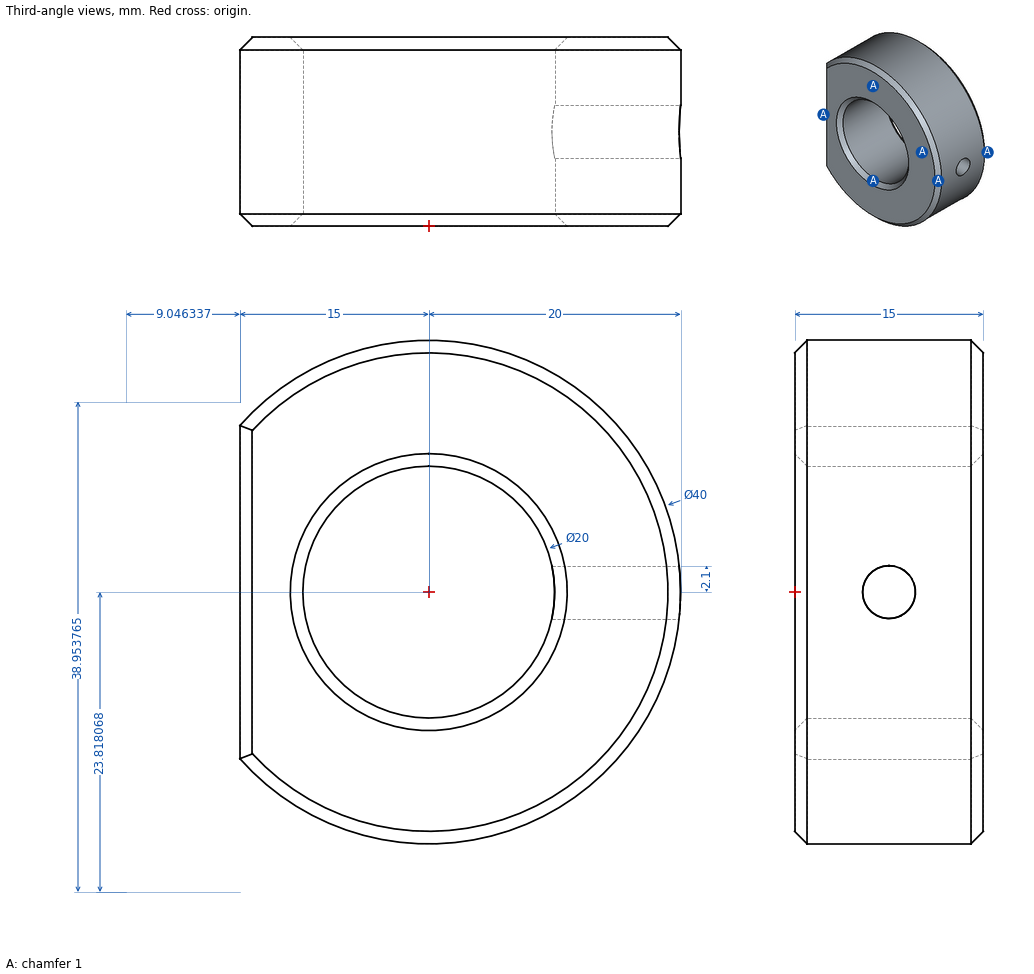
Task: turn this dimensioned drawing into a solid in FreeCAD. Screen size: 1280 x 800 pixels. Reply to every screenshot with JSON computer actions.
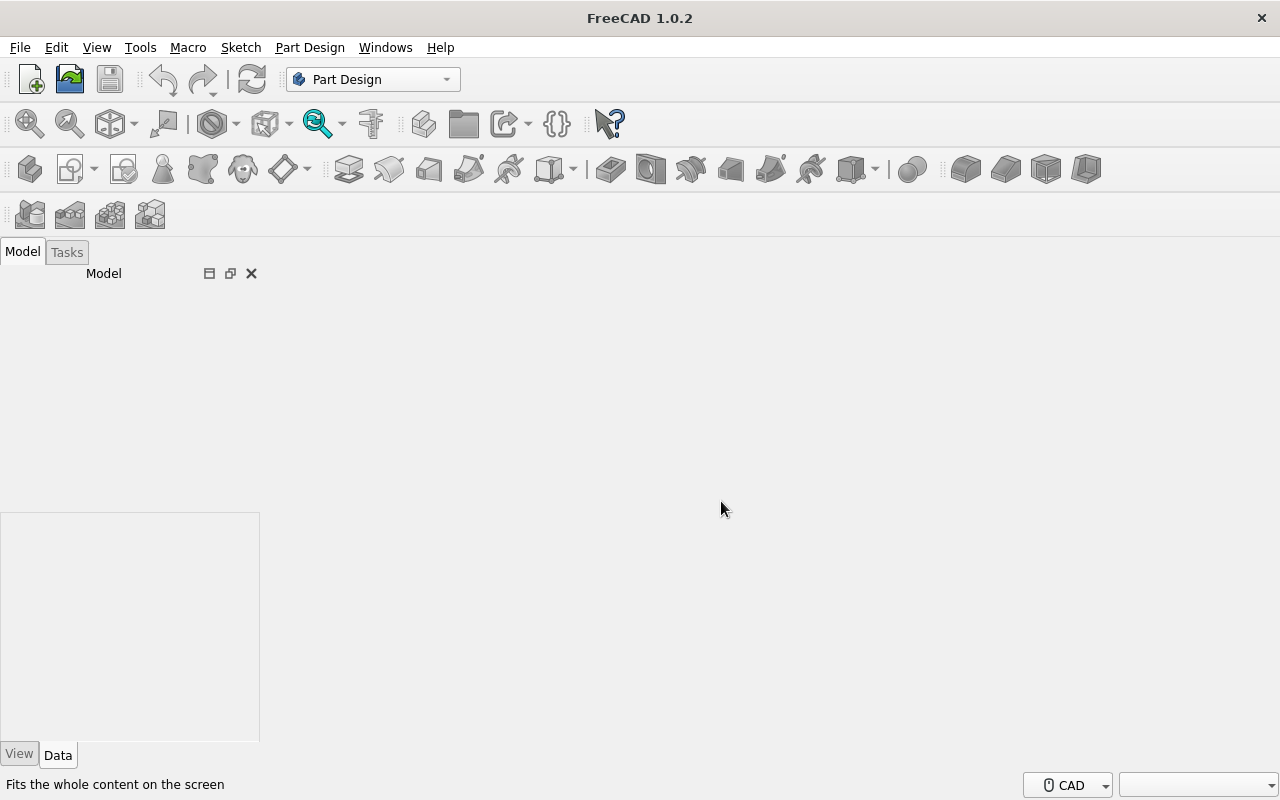
{"action": "key", "text": "ctrl+n"}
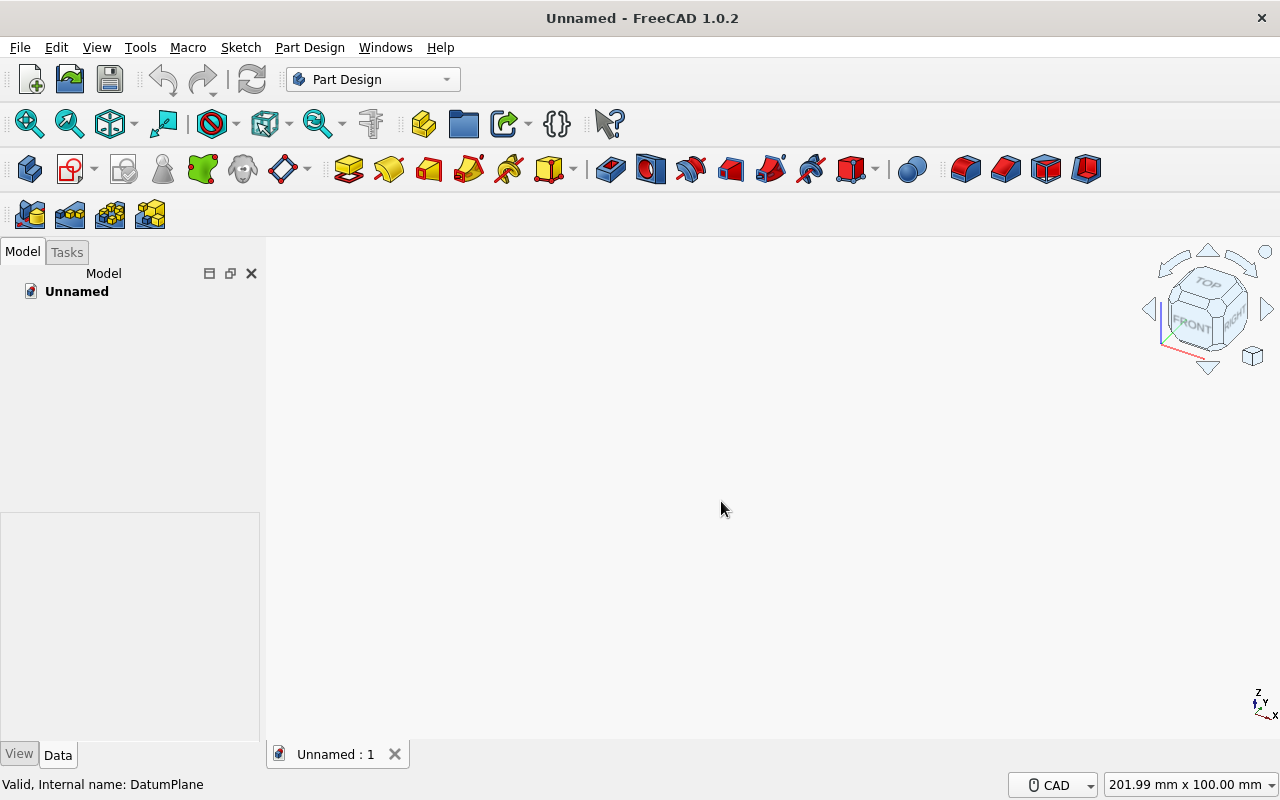
{"action": "left_click", "coordinate": [70, 170]}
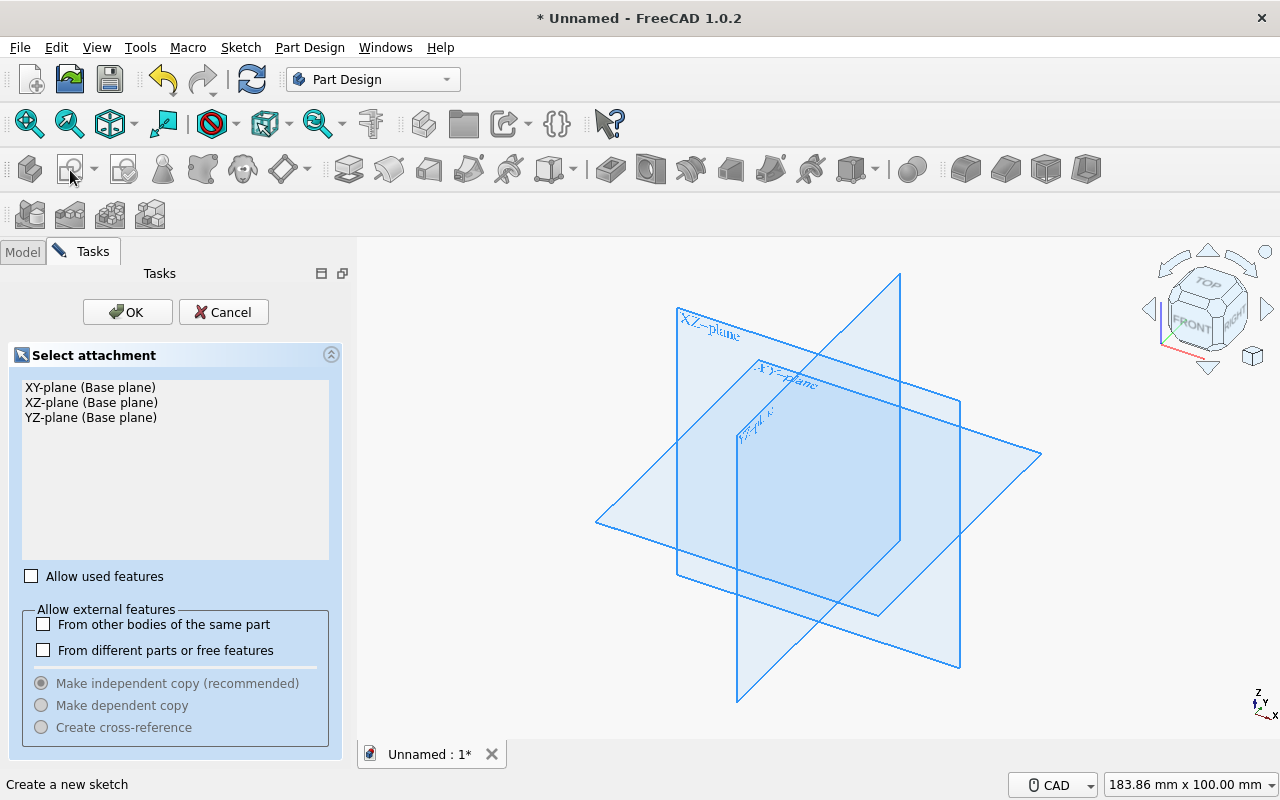
{"action": "left_click", "coordinate": [82, 402]}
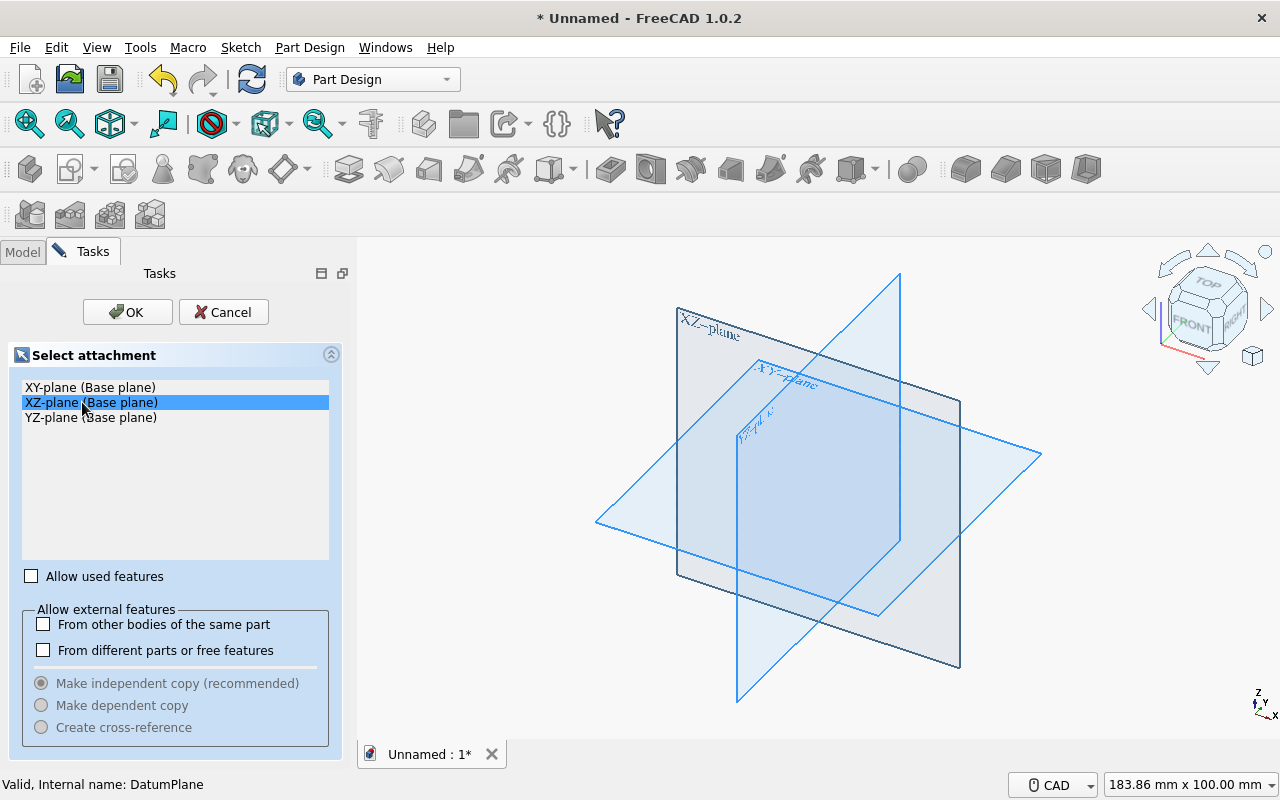
{"action": "left_click", "coordinate": [128, 312]}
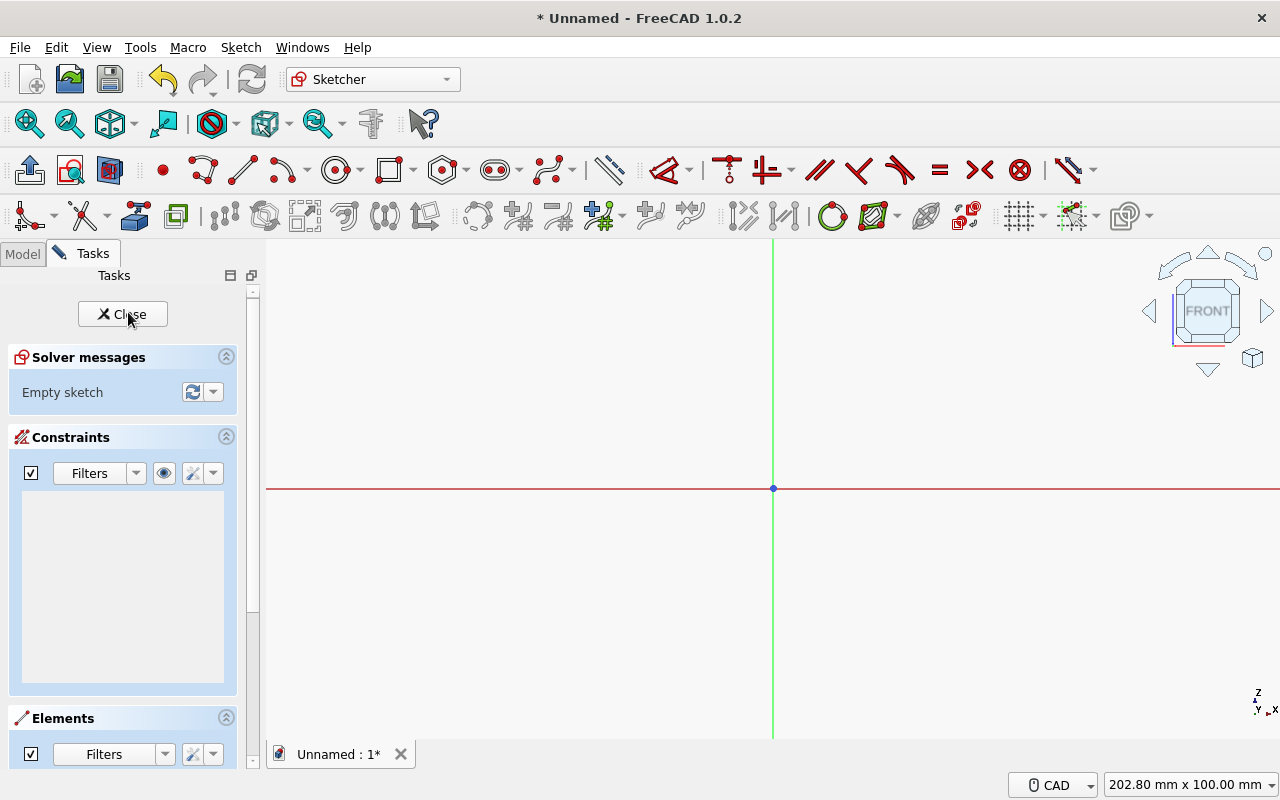
{"action": "scroll", "coordinate": [912, 489], "scroll_direction": "up", "scroll_amount": 2}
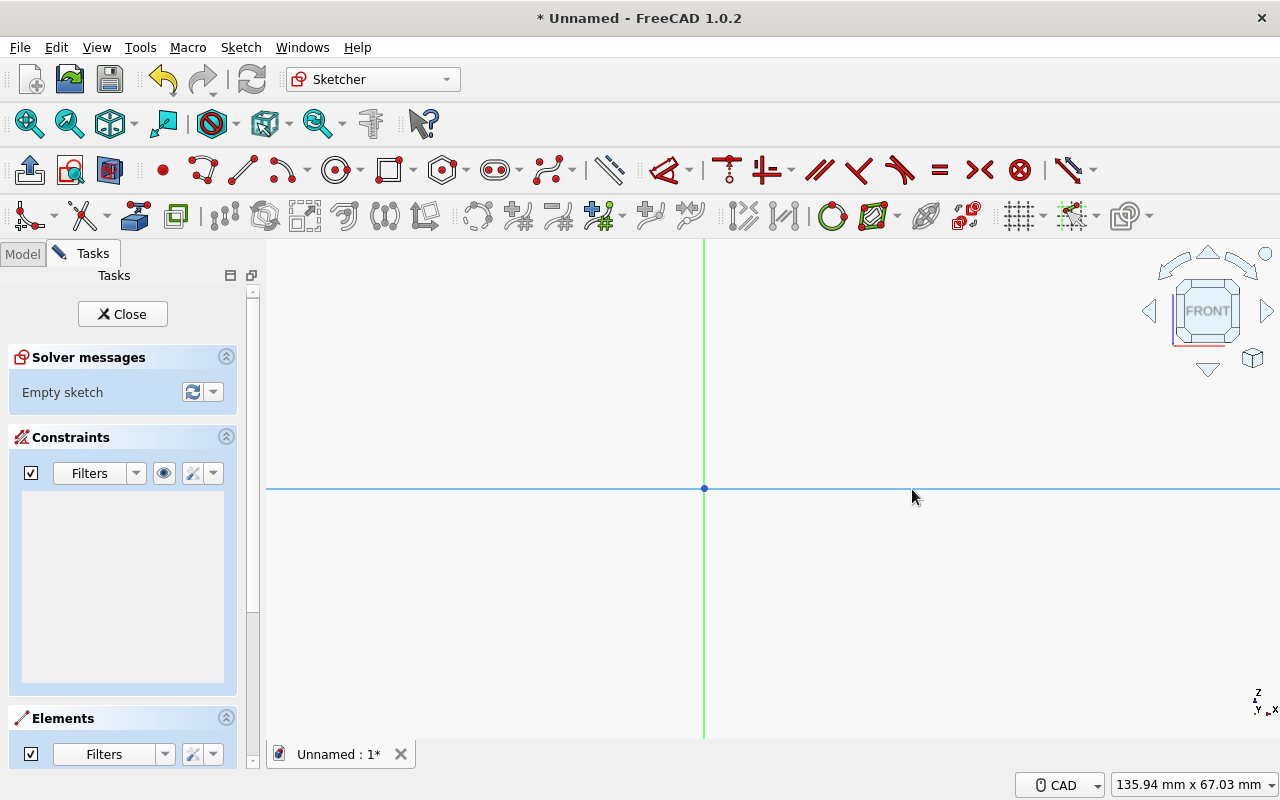
{"action": "key", "text": "g c"}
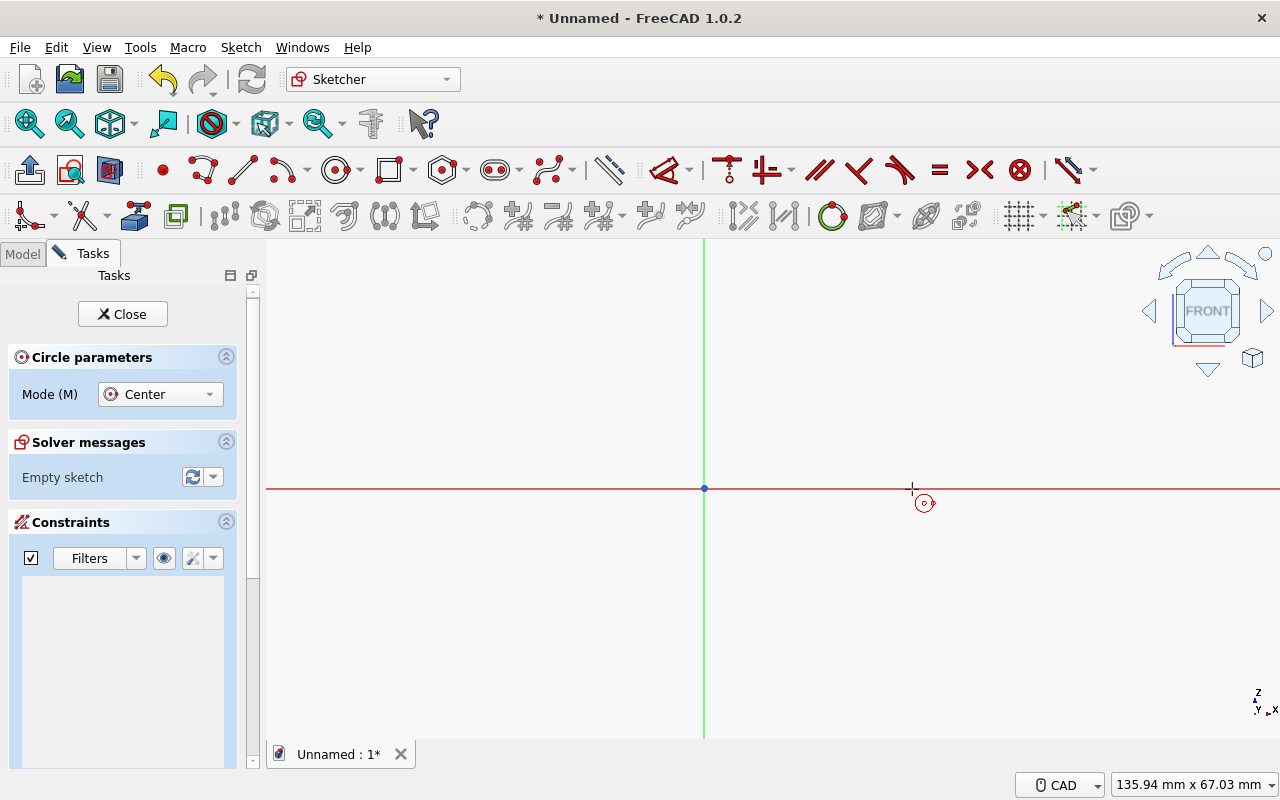
{"action": "left_click", "coordinate": [704, 489]}
{"action": "mouse_move", "coordinate": [810, 383]}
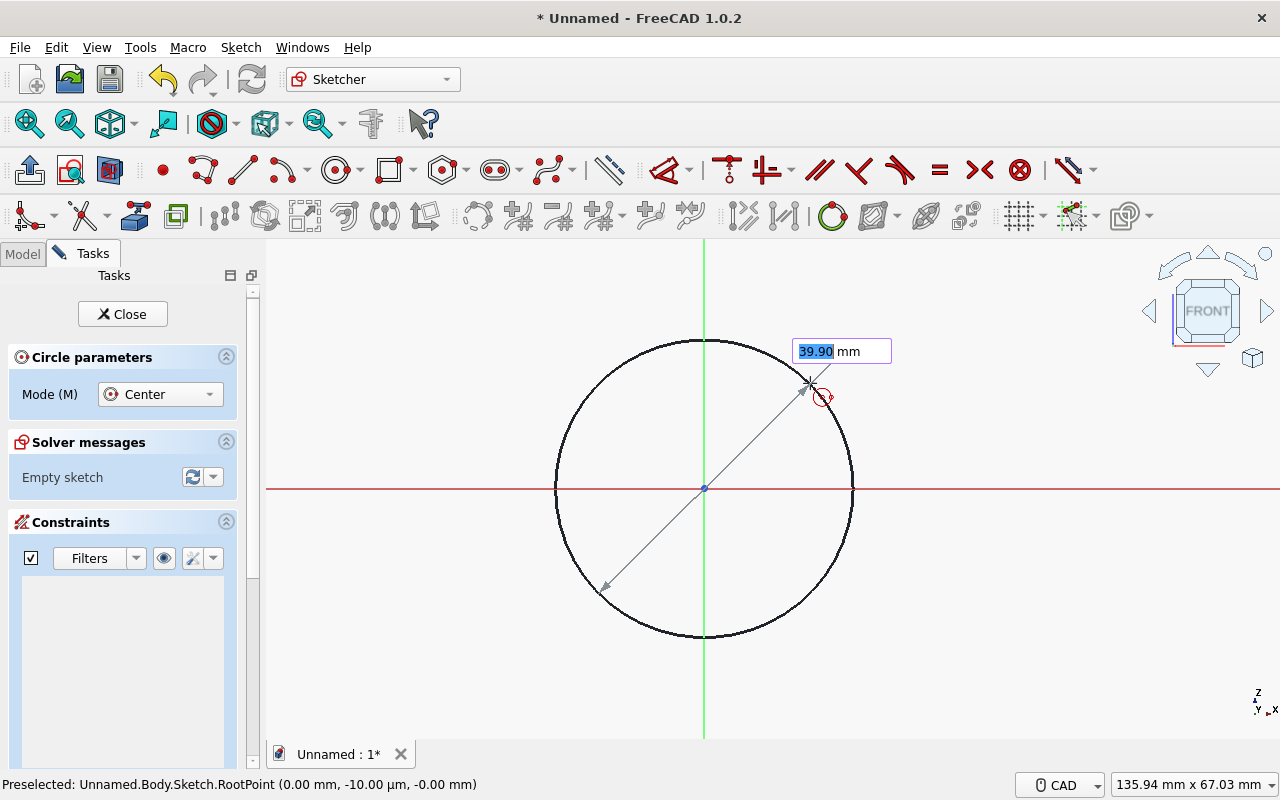
{"action": "type", "text": "40"}
{"action": "key", "text": "Return"}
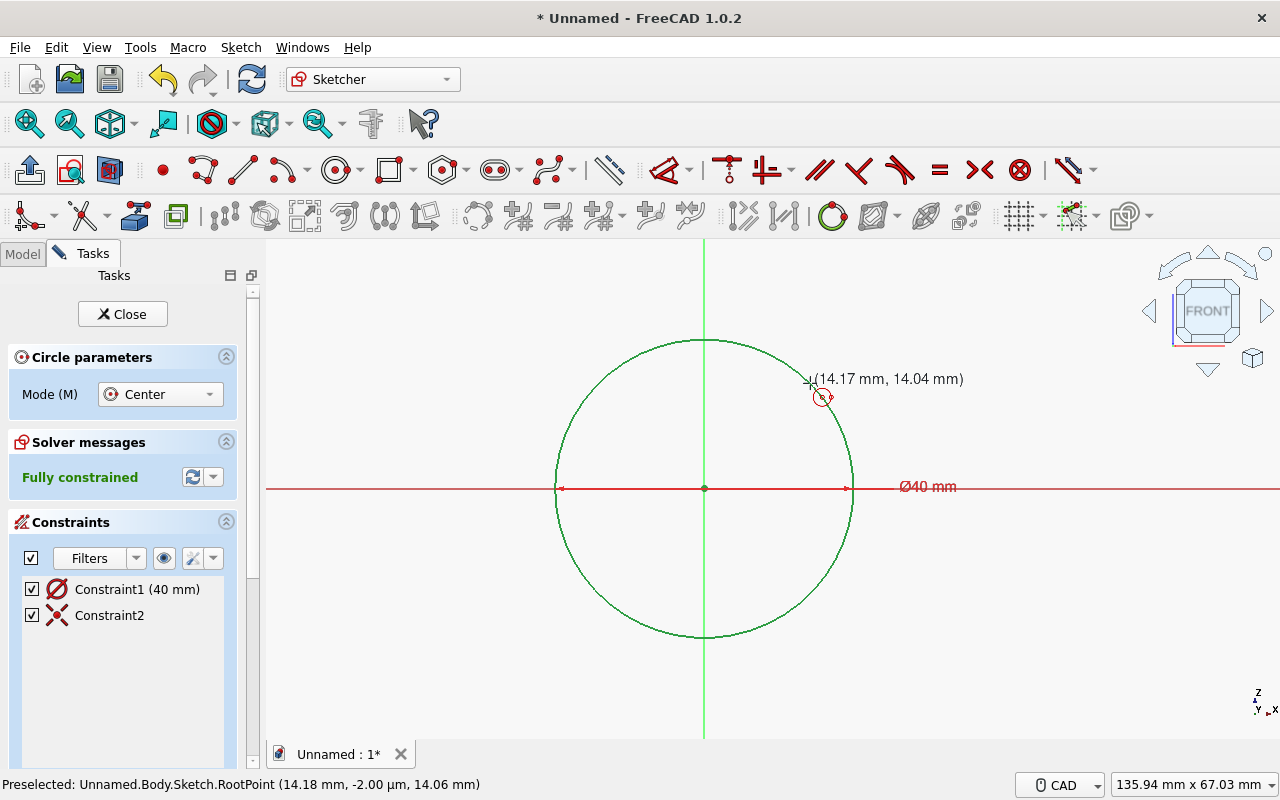
{"action": "left_click", "coordinate": [704, 489]}
{"action": "mouse_move", "coordinate": [757, 436]}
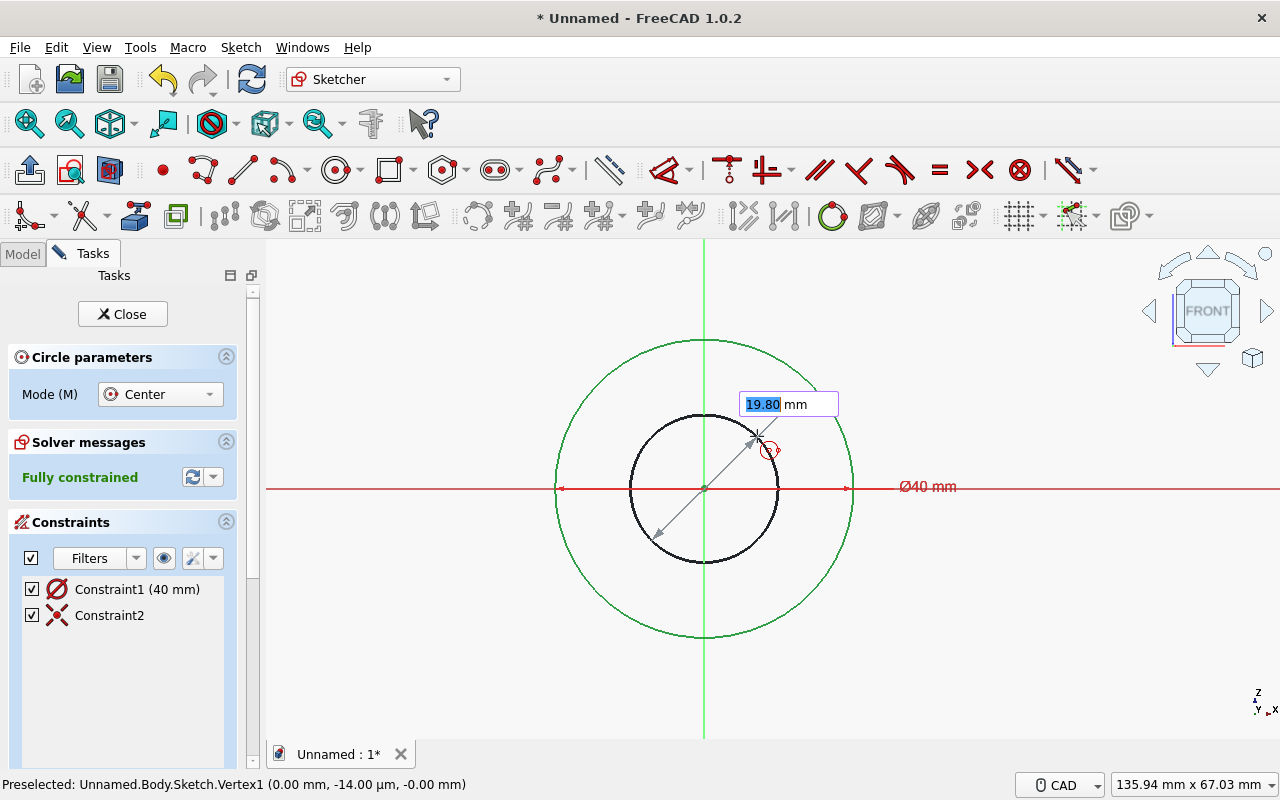
{"action": "type", "text": "20"}
{"action": "key", "text": "Return"}
{"action": "key", "text": "Escape"}